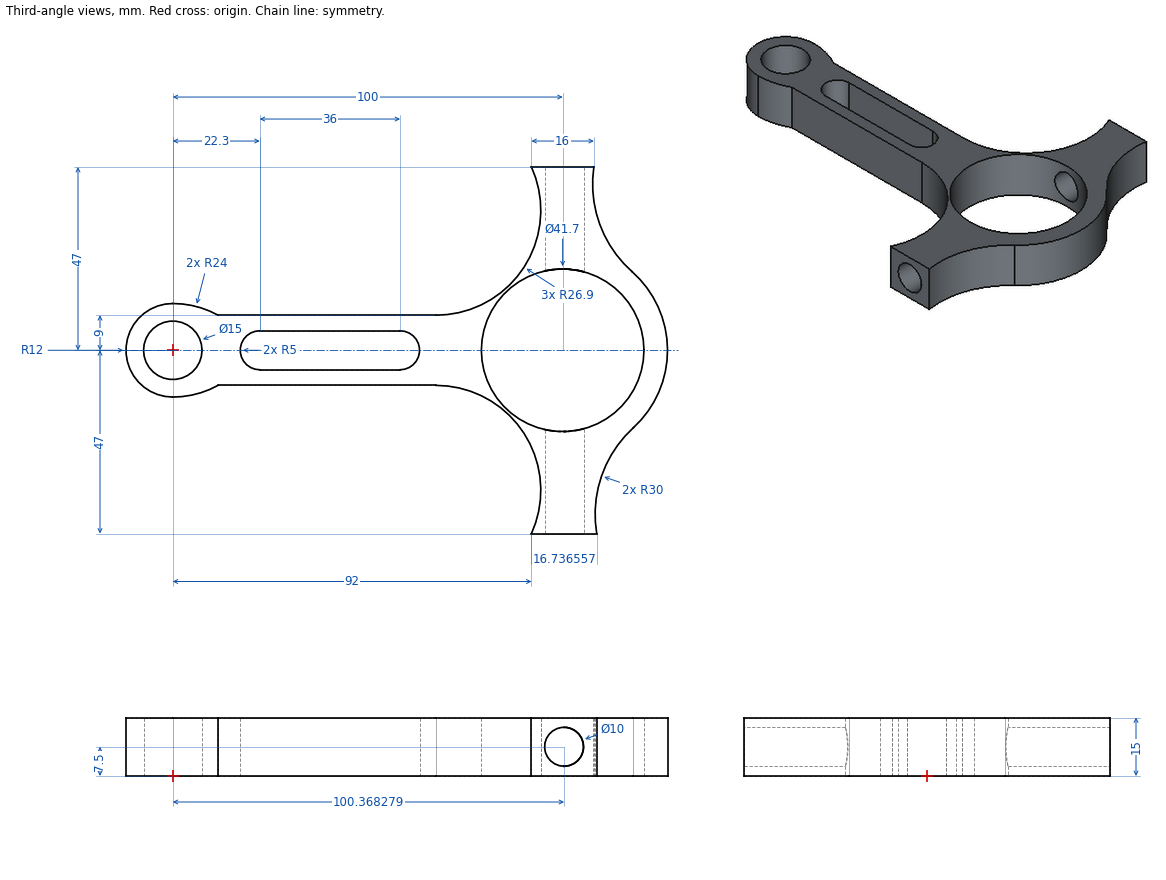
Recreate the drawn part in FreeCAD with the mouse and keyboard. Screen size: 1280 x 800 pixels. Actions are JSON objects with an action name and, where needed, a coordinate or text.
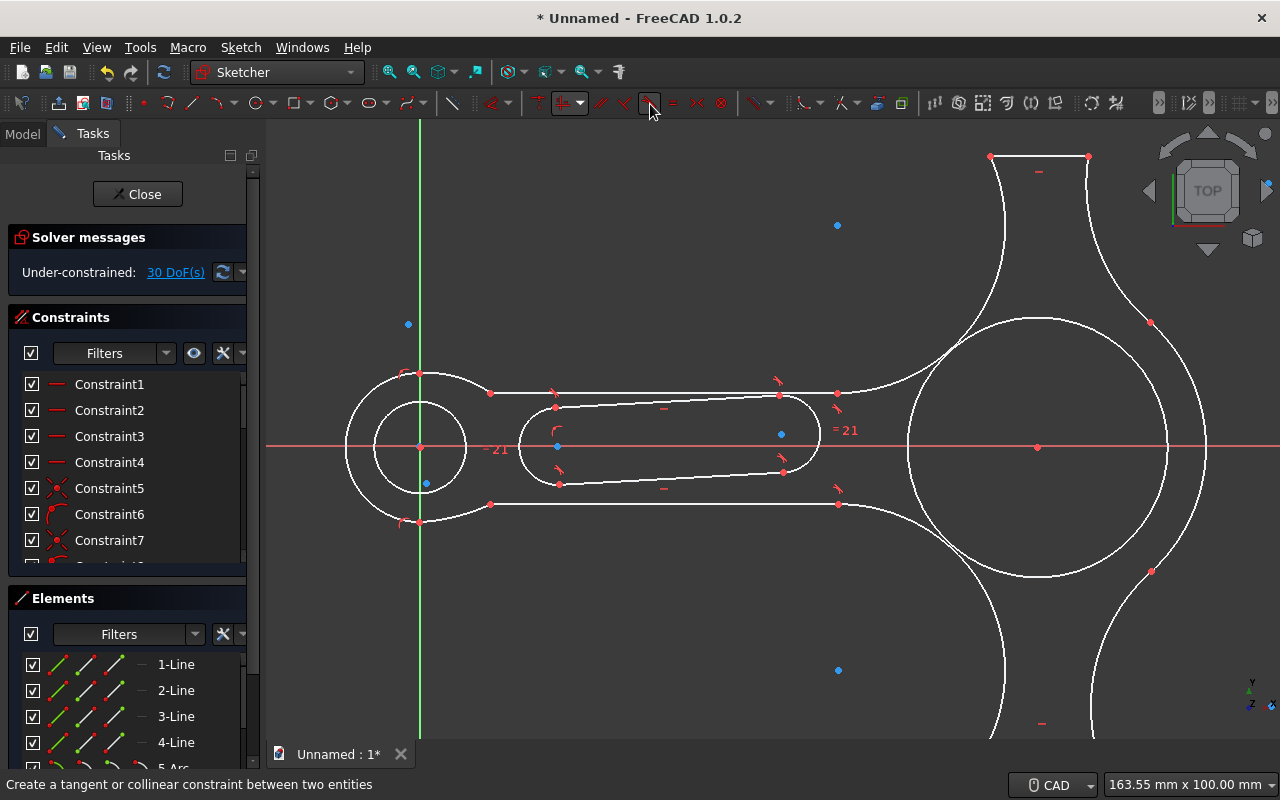
{"action": "left_click", "coordinate": [471, 382]}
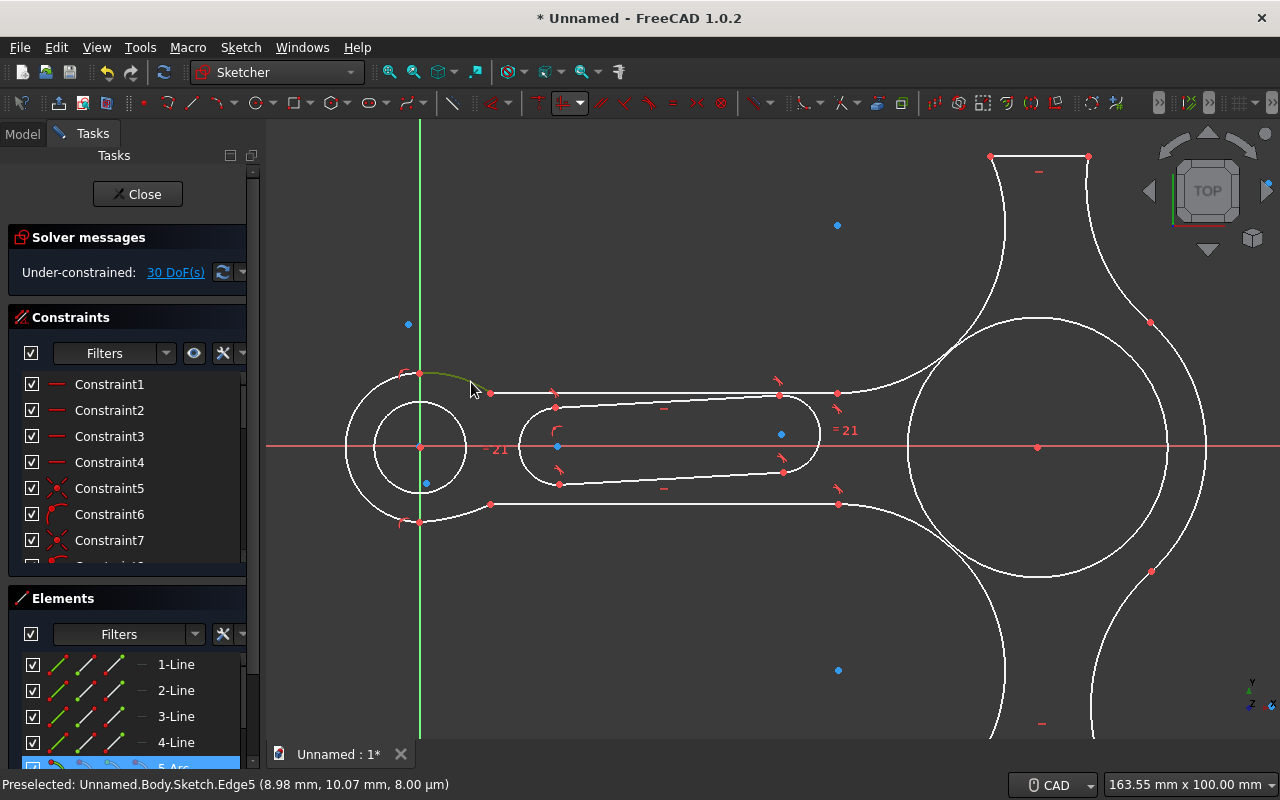
{"action": "left_click", "coordinate": [360, 404]}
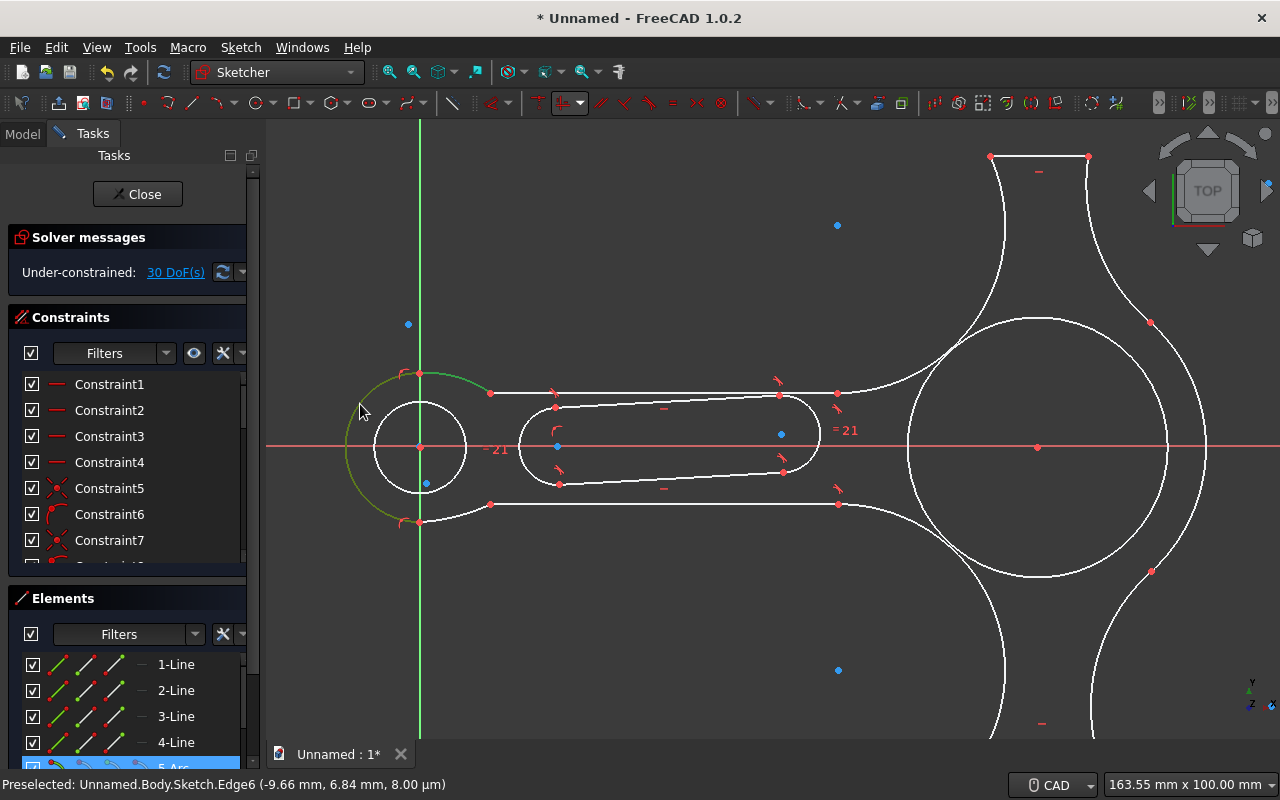
{"action": "left_click", "coordinate": [650, 104]}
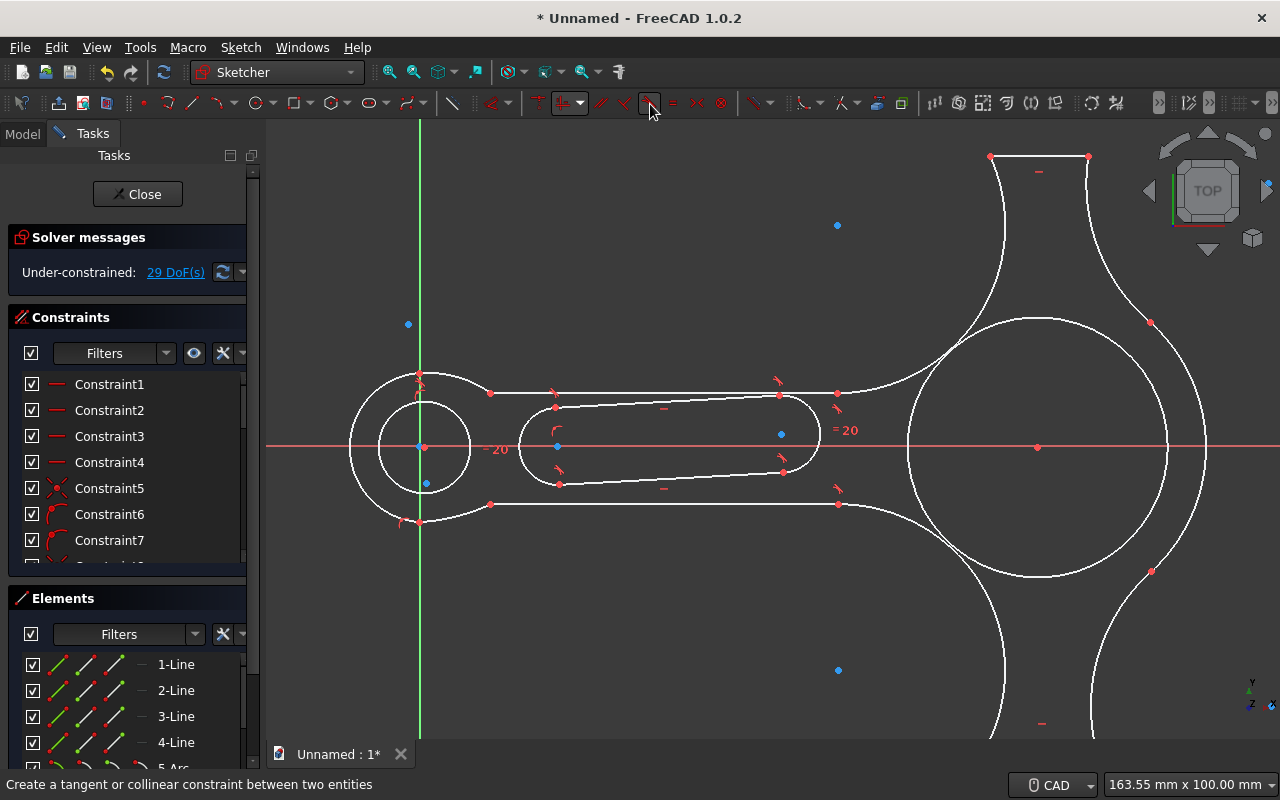
{"action": "left_click", "coordinate": [363, 405]}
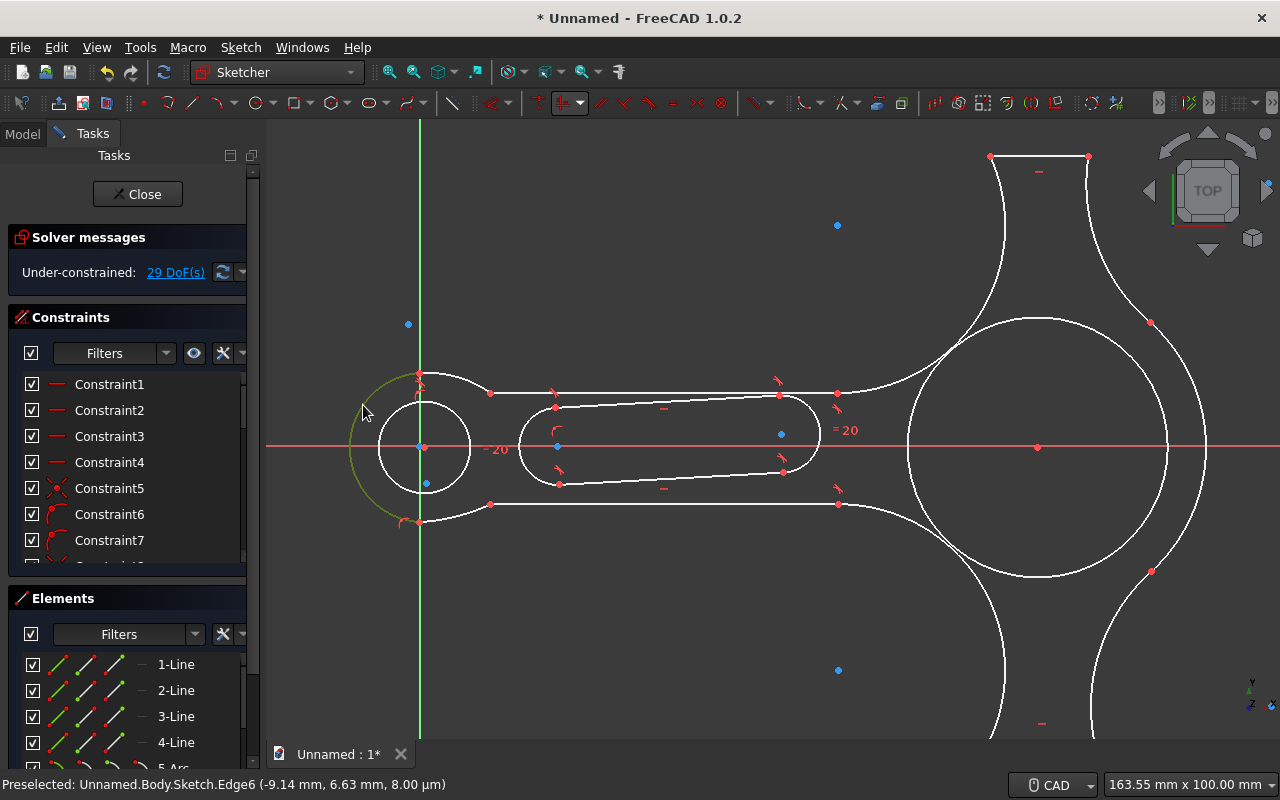
{"action": "left_click", "coordinate": [442, 520]}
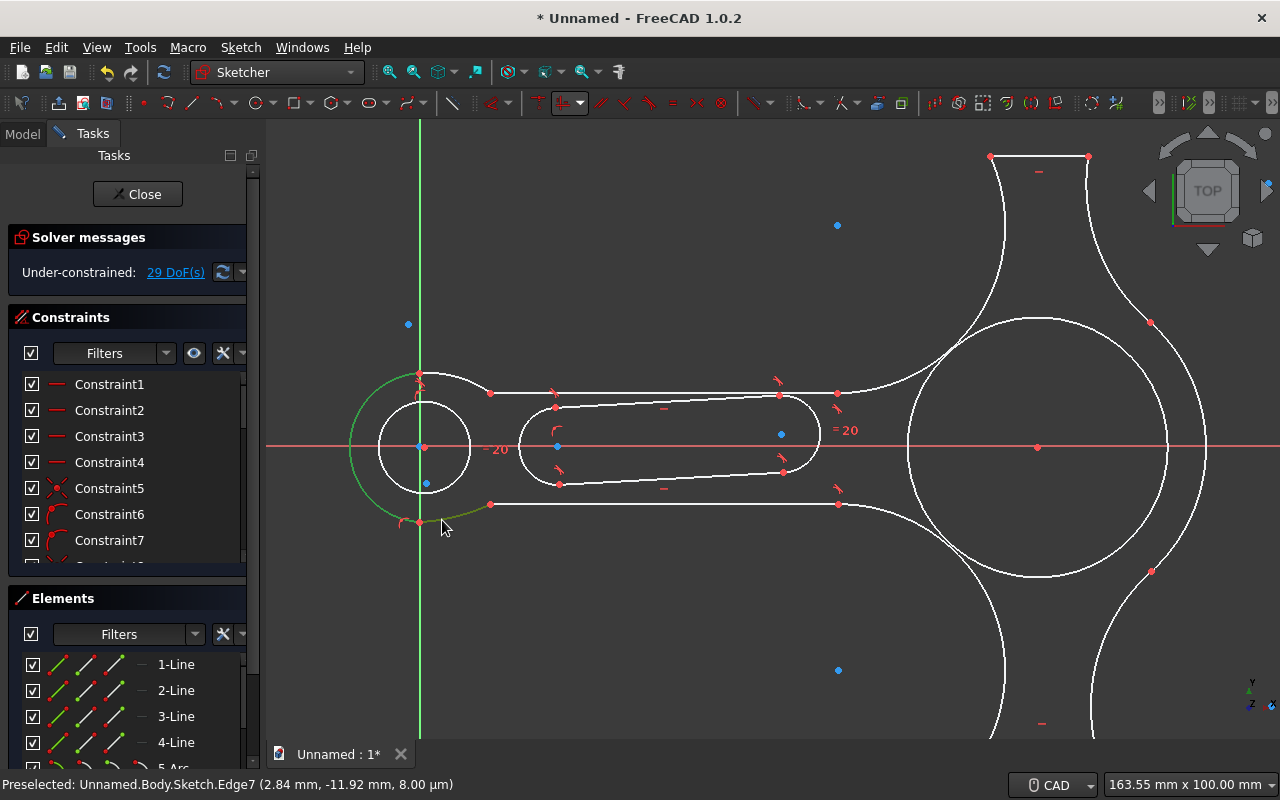
{"action": "left_click", "coordinate": [650, 104]}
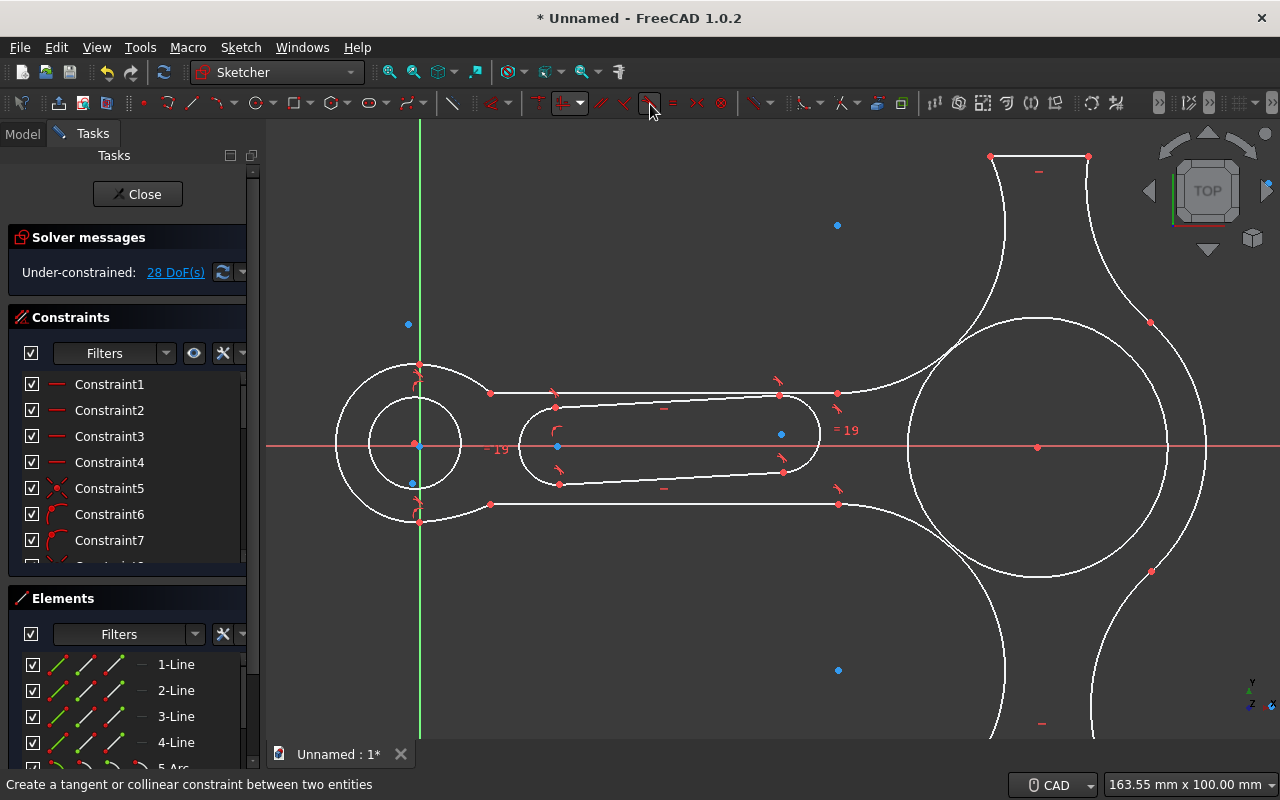
{"action": "left_click", "coordinate": [1092, 684]}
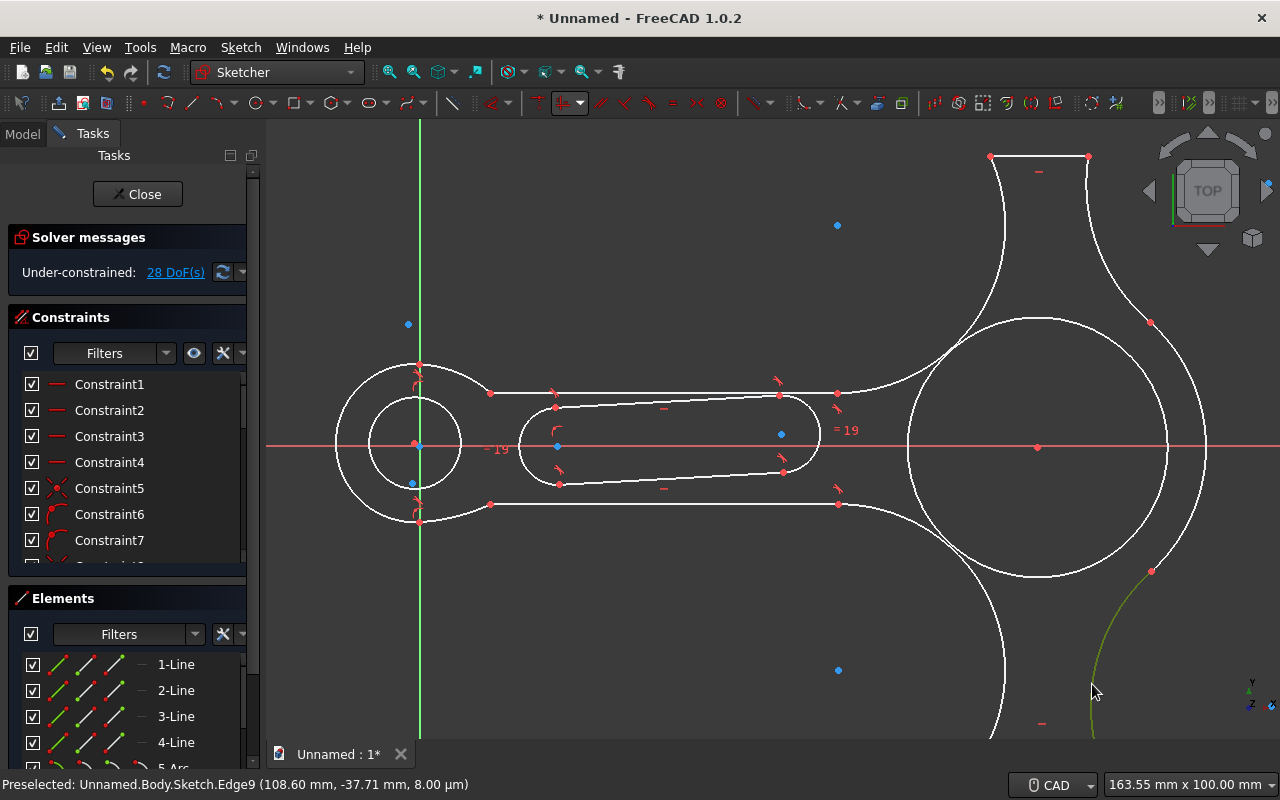
{"action": "scroll", "coordinate": [560, 394], "scroll_direction": "down", "scroll_amount": 2}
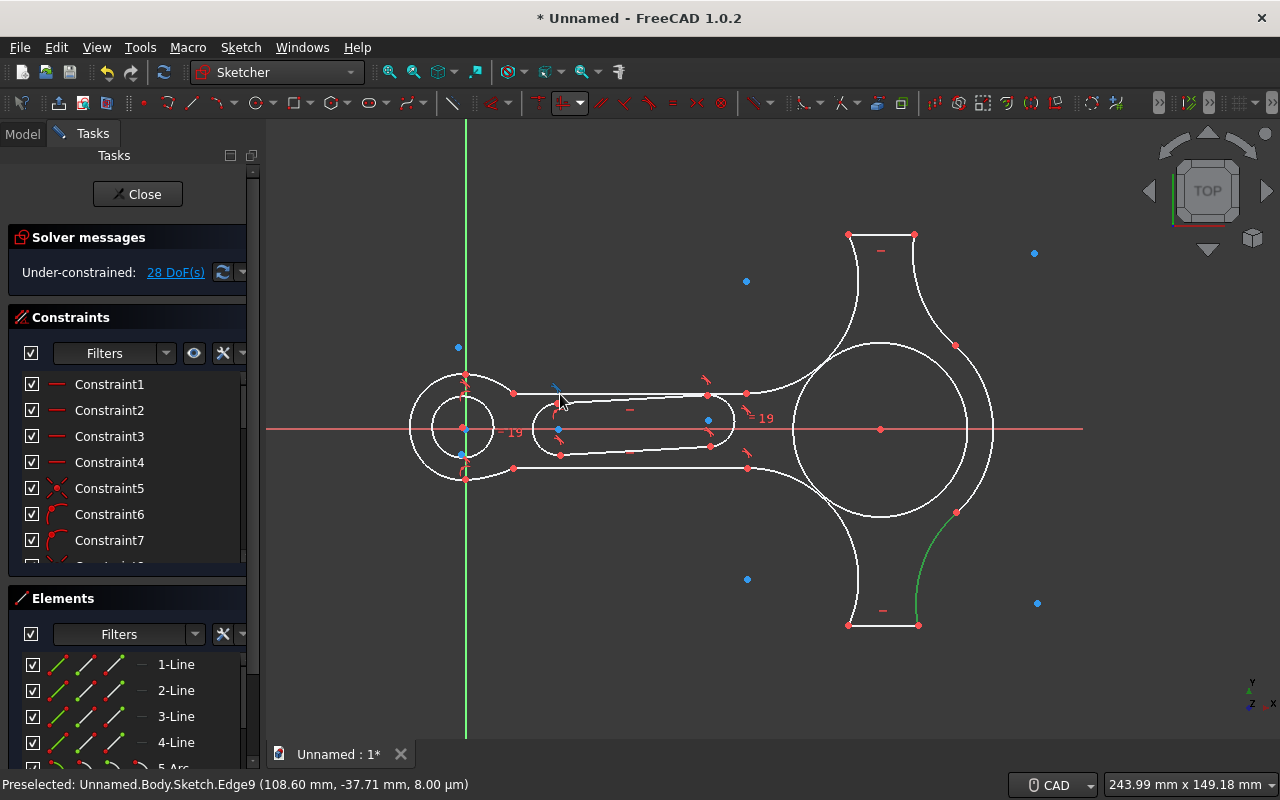
{"action": "left_click", "coordinate": [987, 466]}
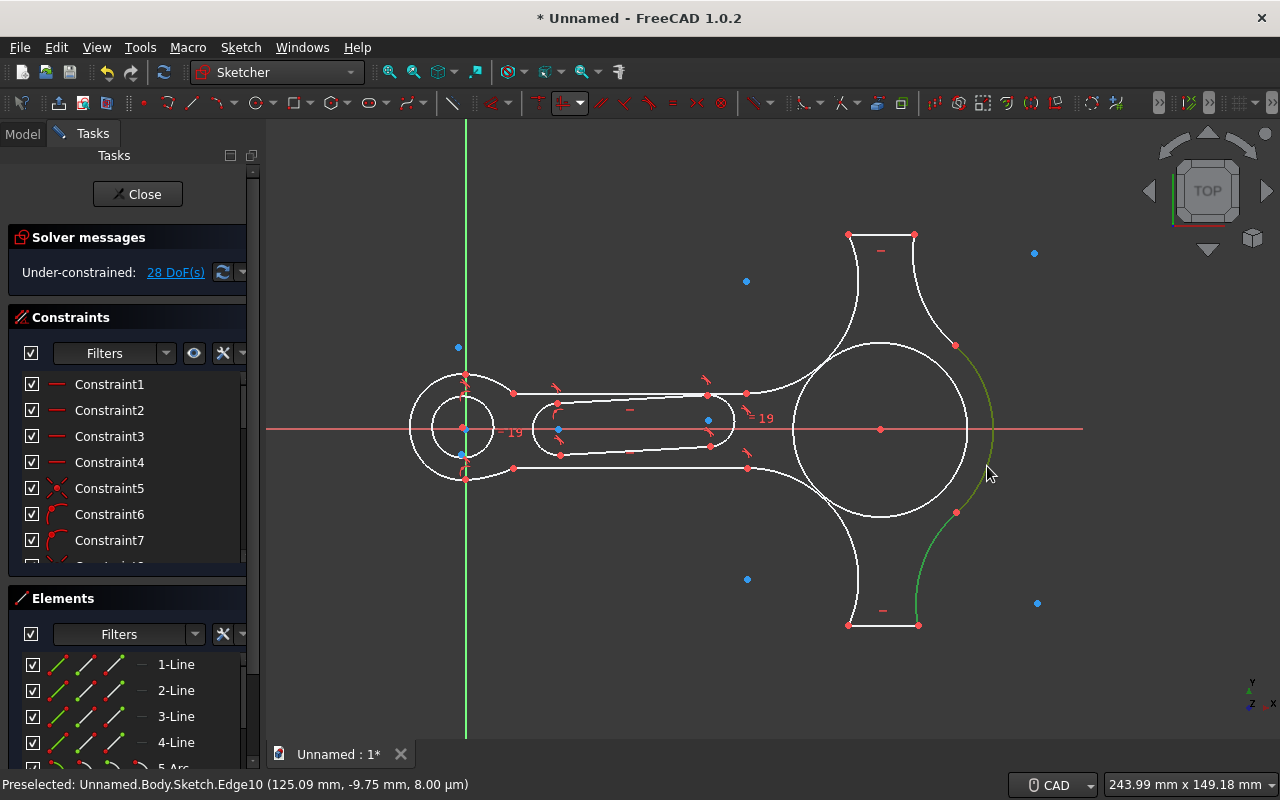
{"action": "left_click", "coordinate": [650, 104]}